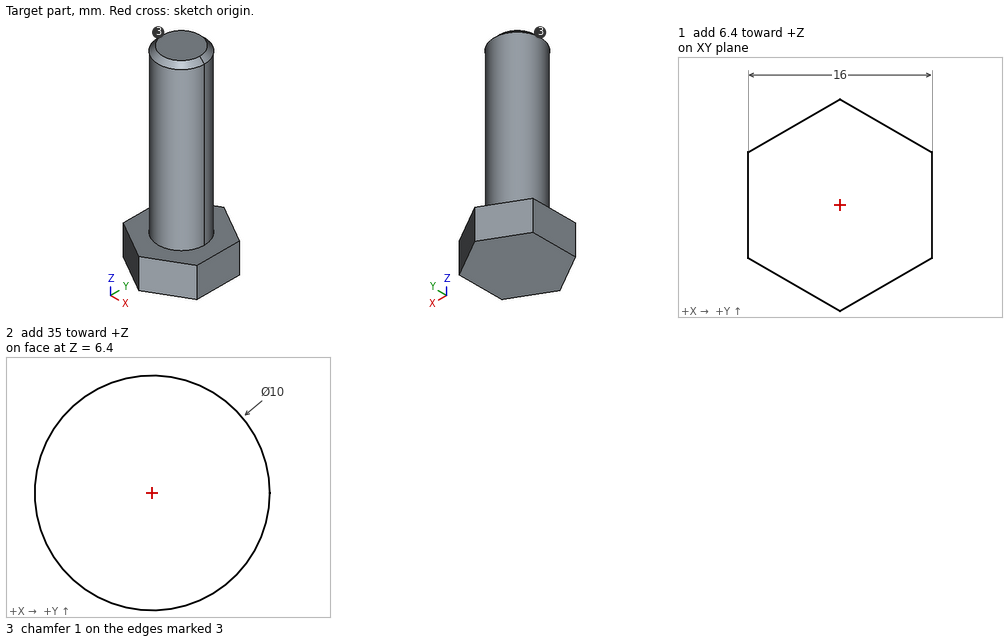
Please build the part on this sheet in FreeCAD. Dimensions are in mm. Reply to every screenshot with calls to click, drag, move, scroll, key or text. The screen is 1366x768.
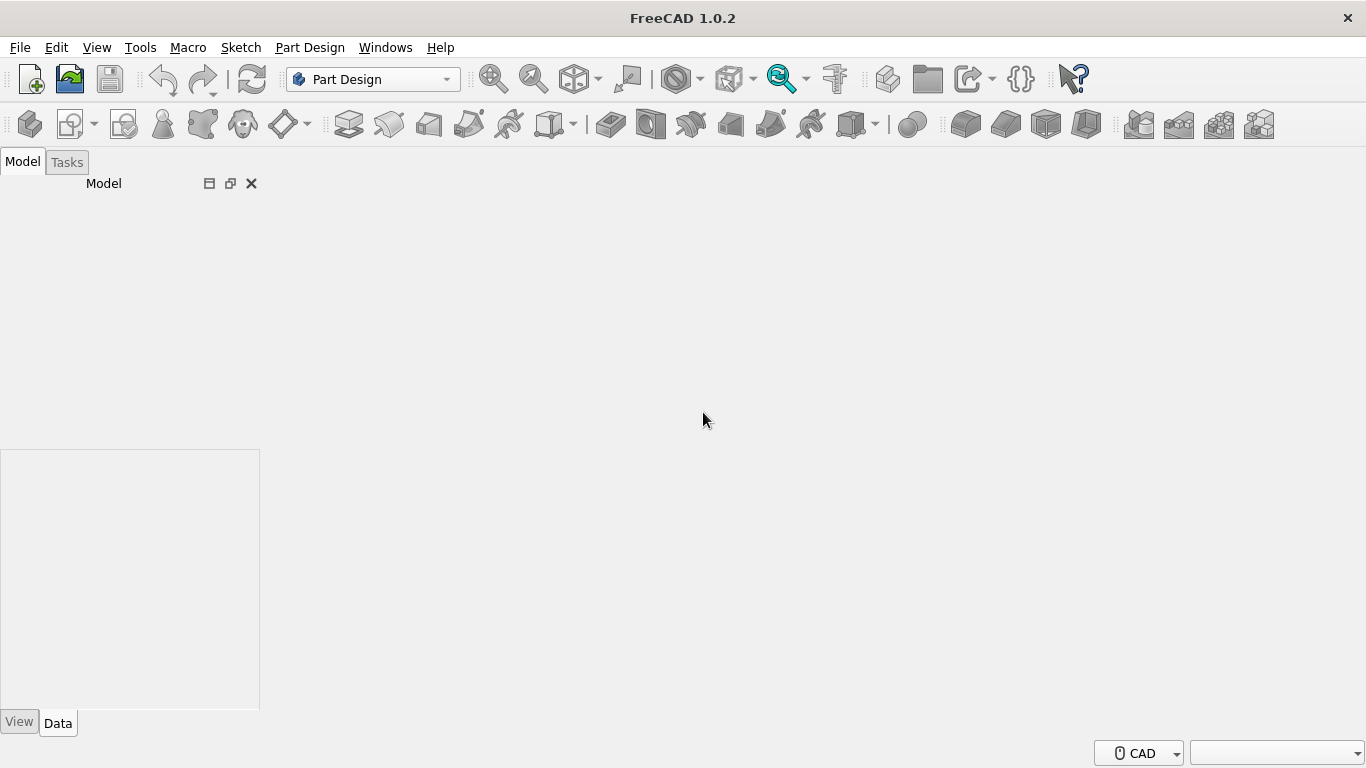
key(ctrl+n)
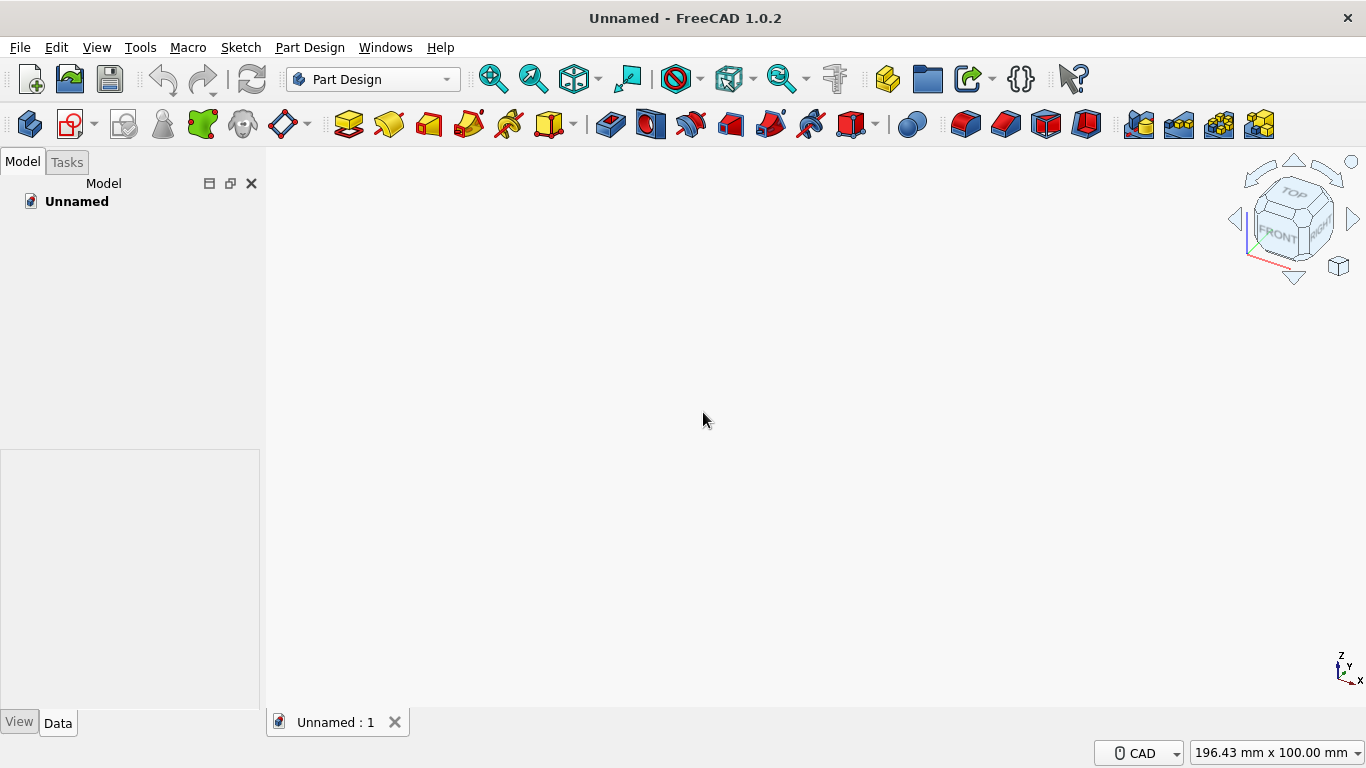
click(70, 124)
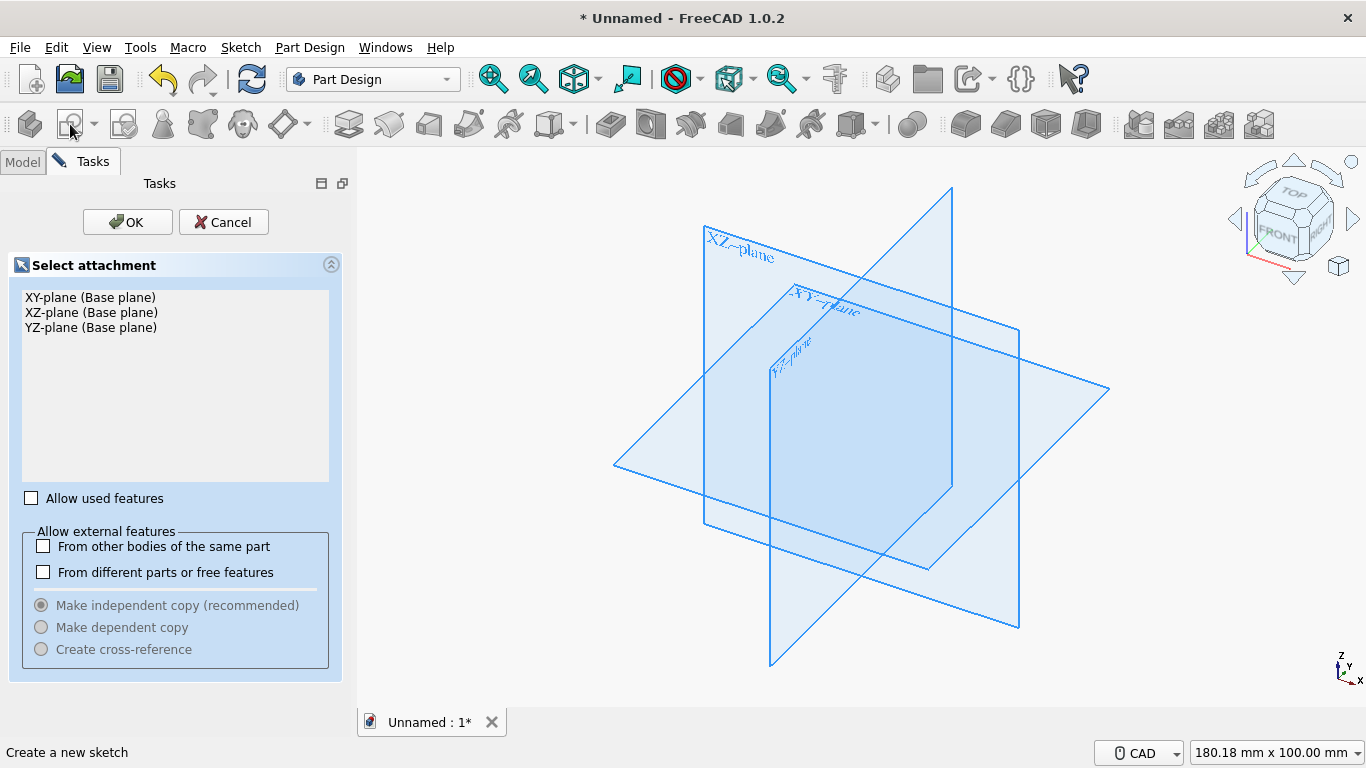
click(82, 298)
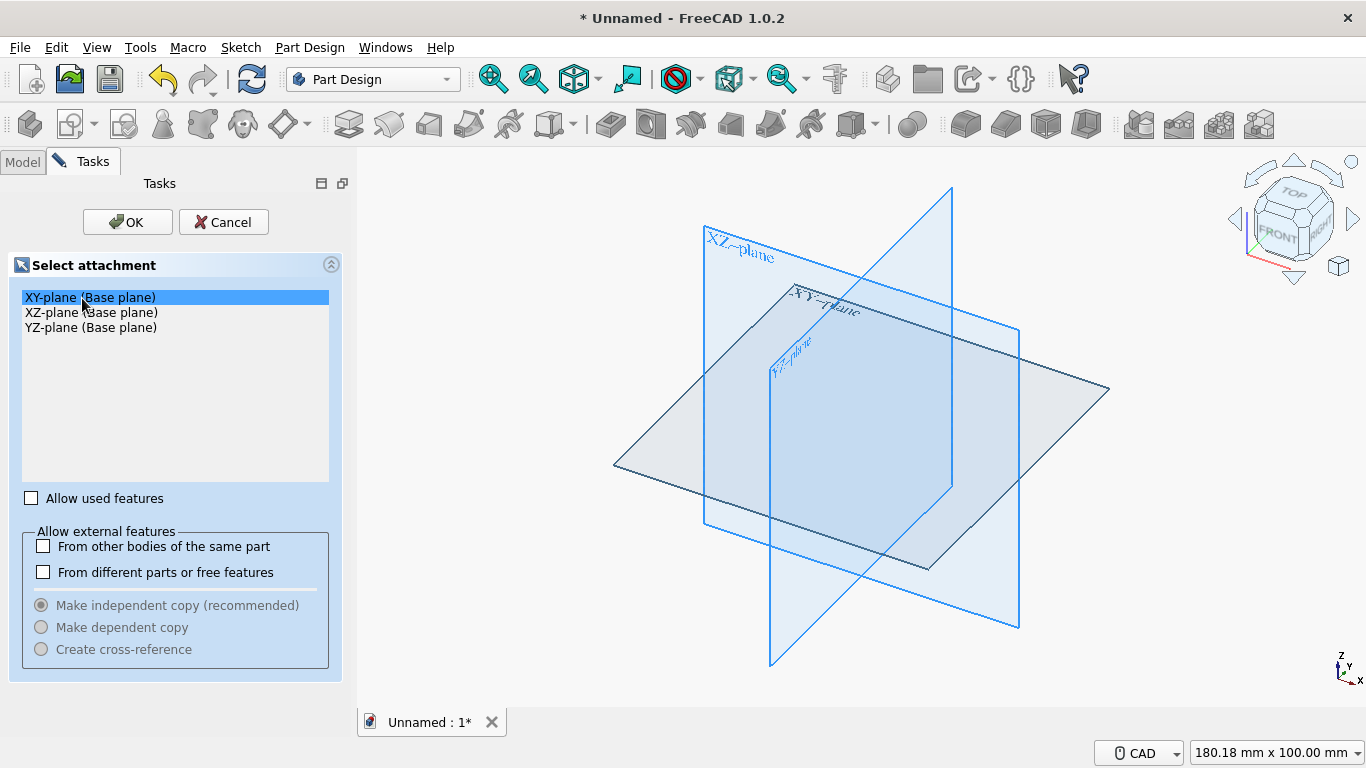
click(128, 222)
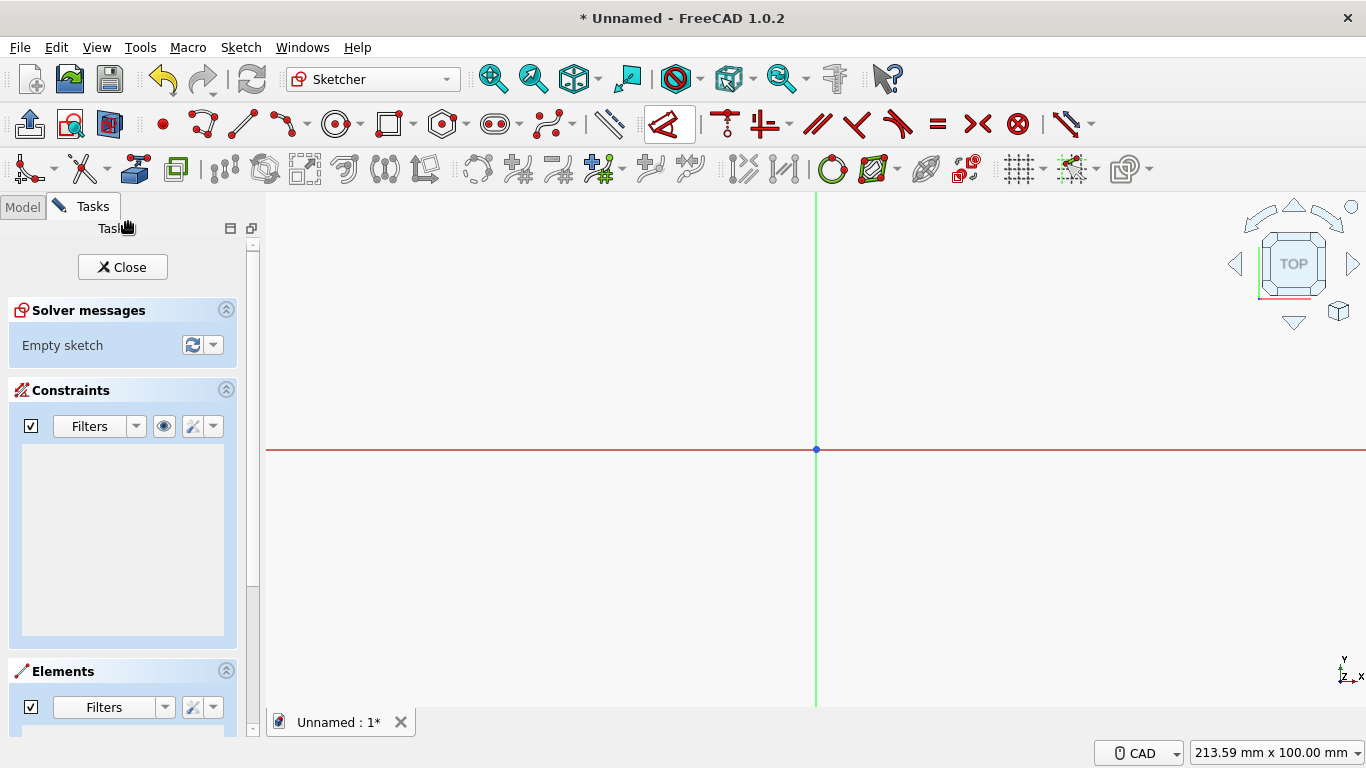
scroll(846, 449, up, 6)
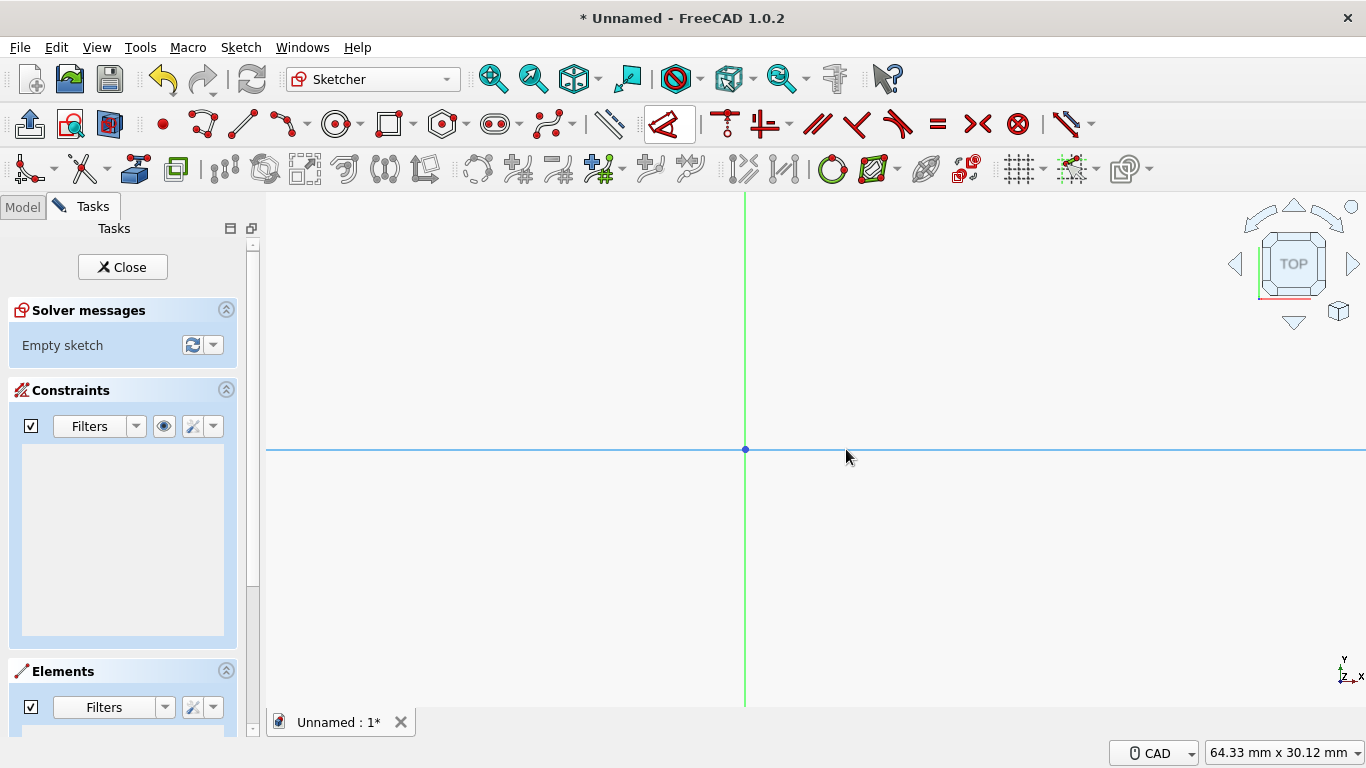
click(442, 124)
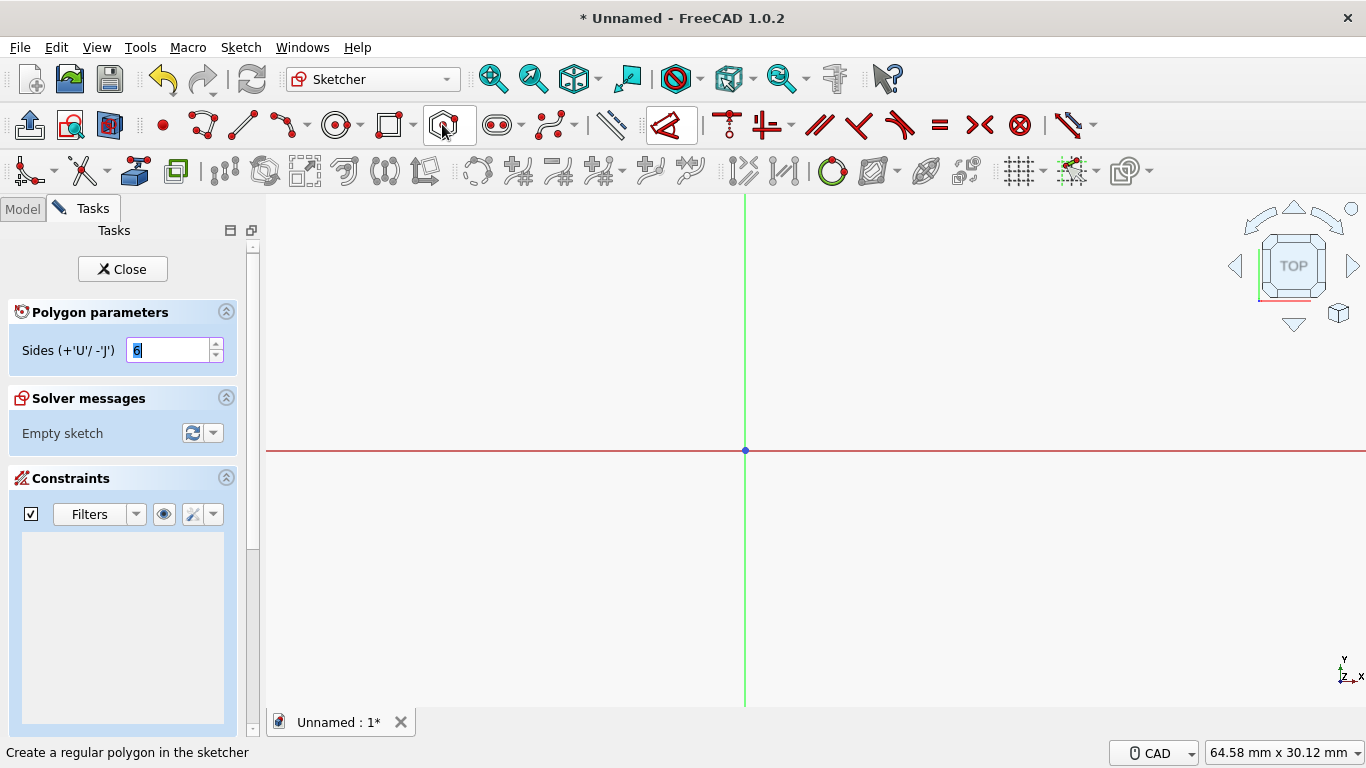
click(745, 450)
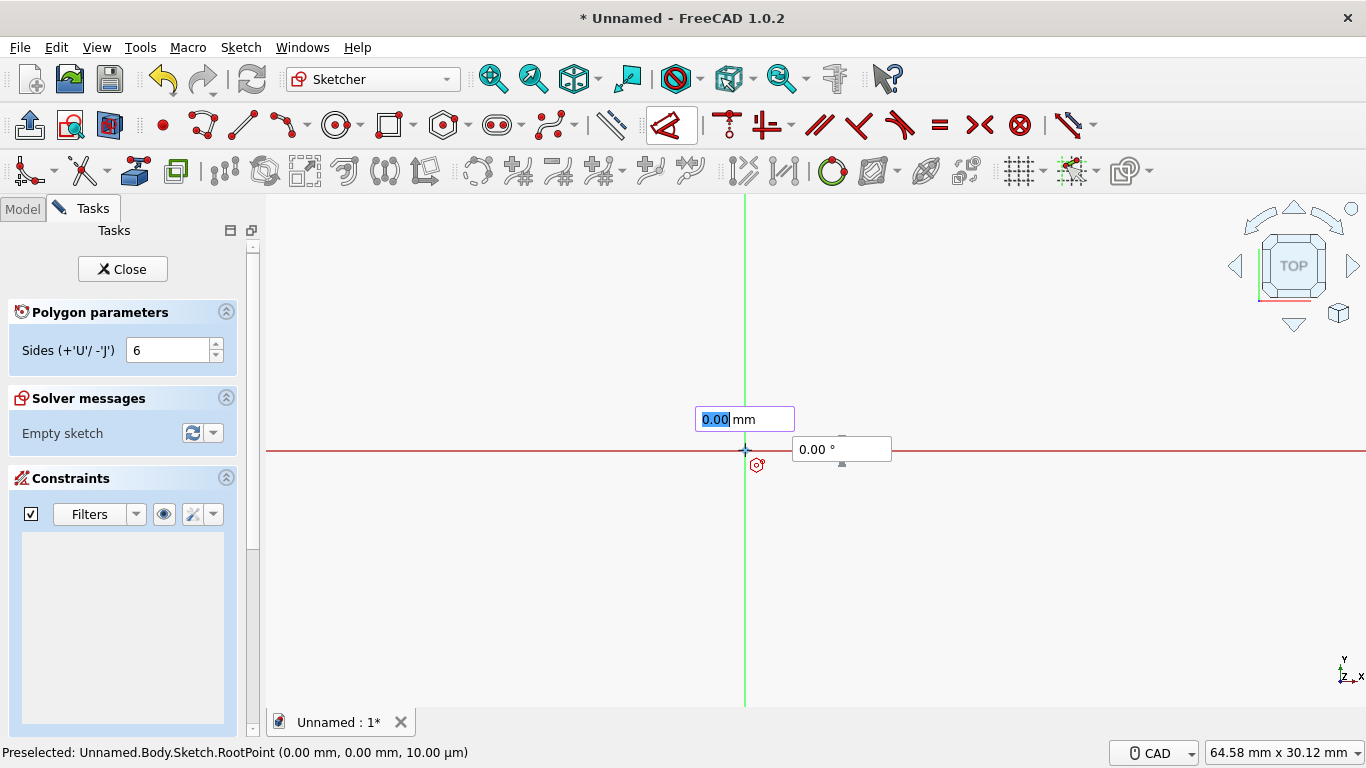
click(745, 293)
right_click(745, 293)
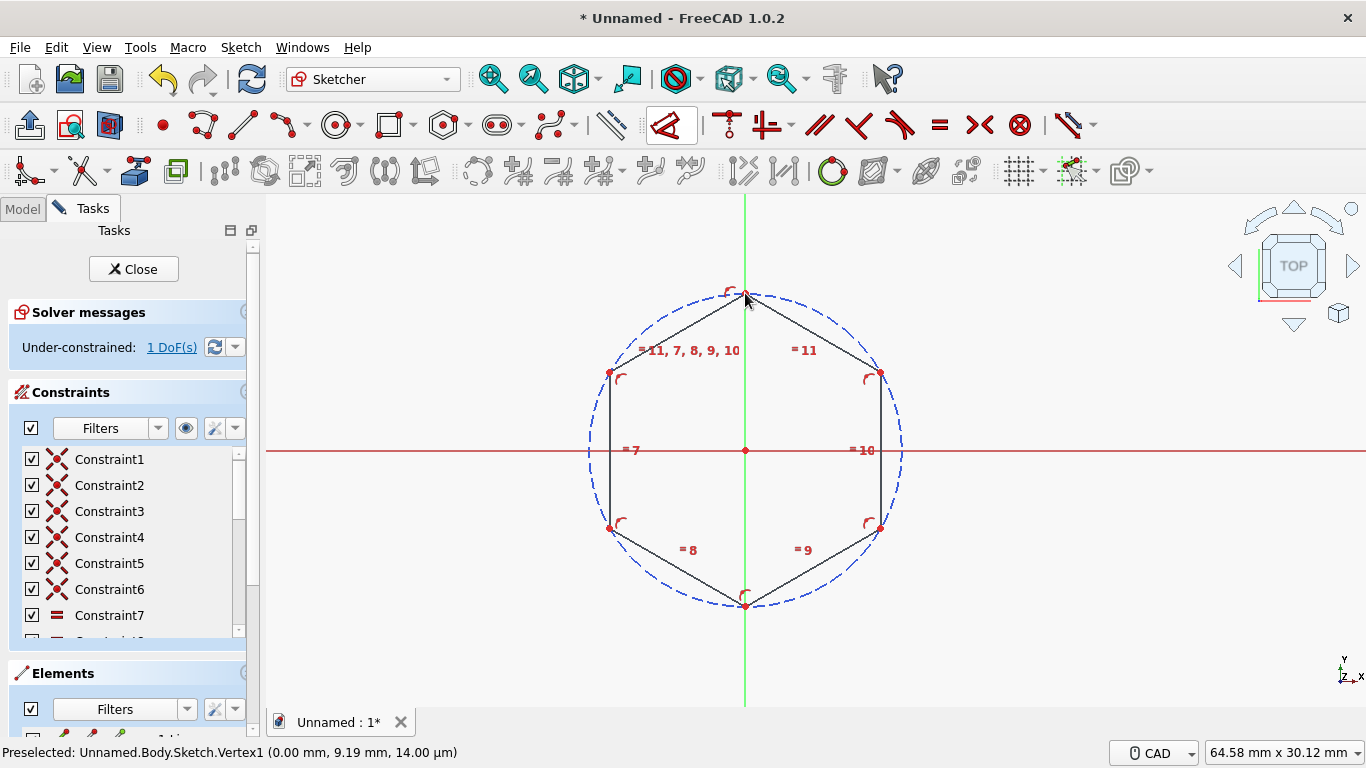
key(d)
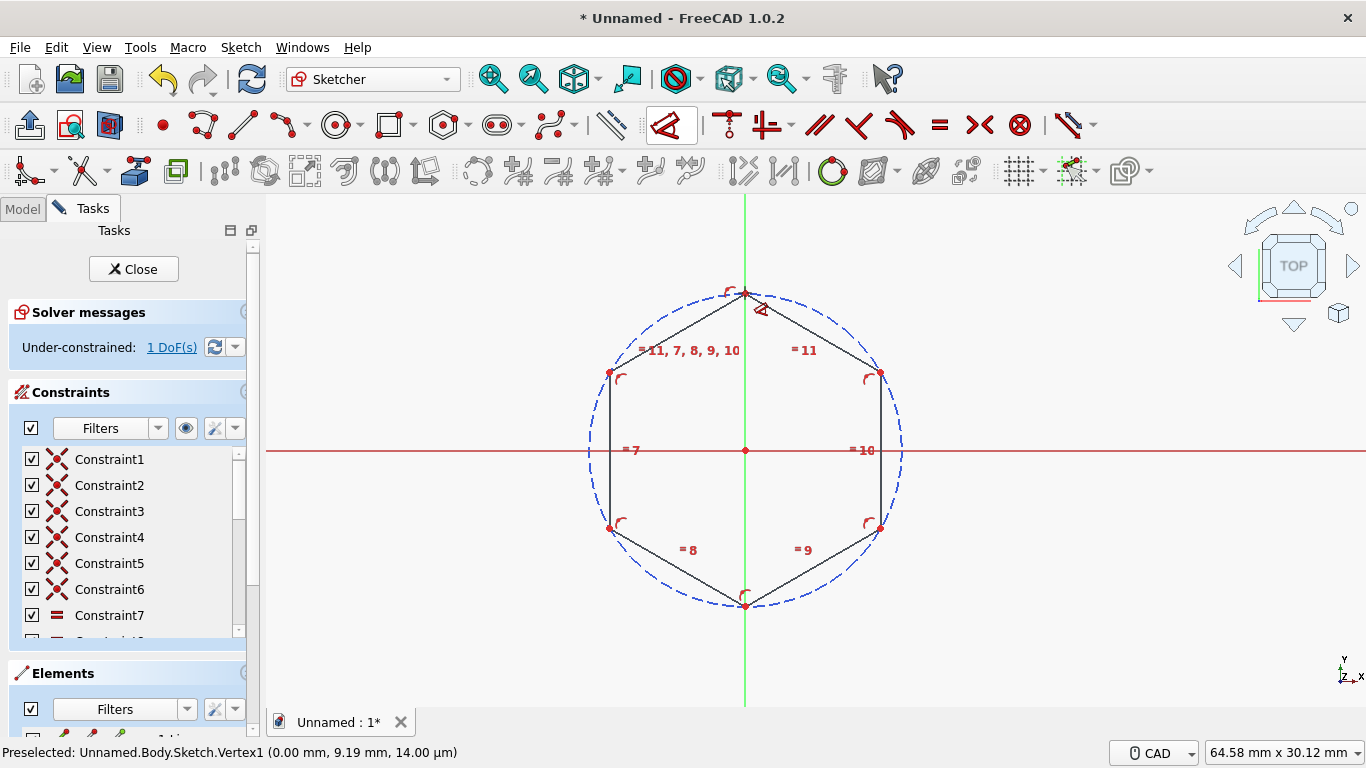
click(610, 372)